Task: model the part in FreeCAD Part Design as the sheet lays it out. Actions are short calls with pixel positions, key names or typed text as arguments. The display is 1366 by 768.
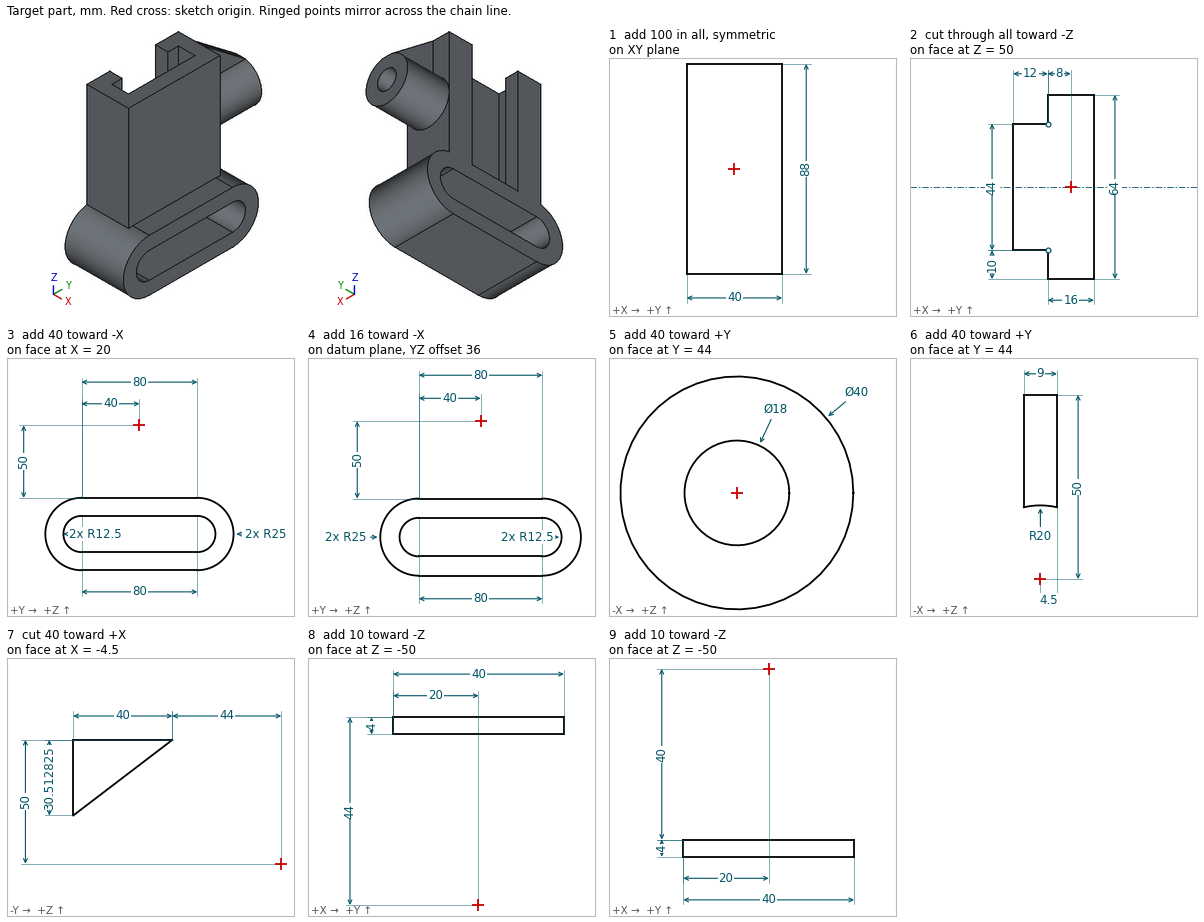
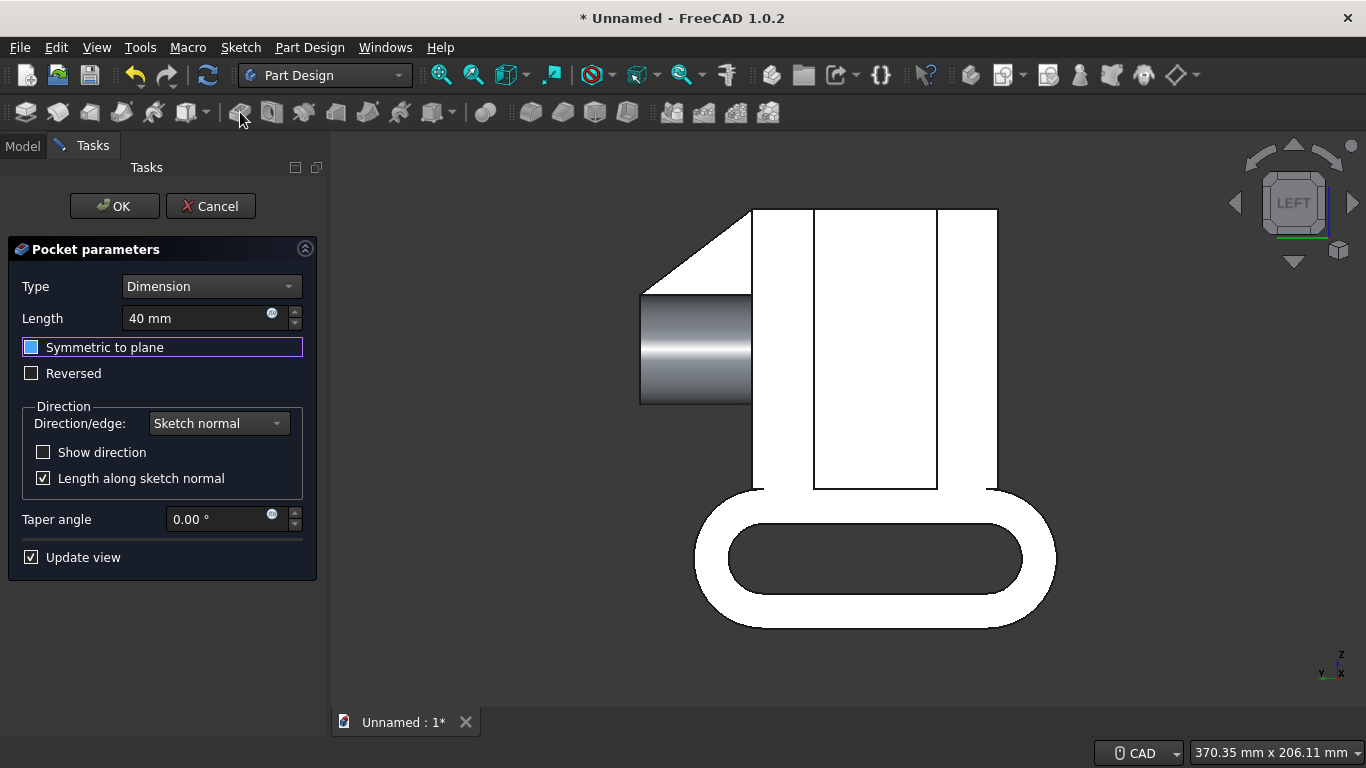
click(115, 206)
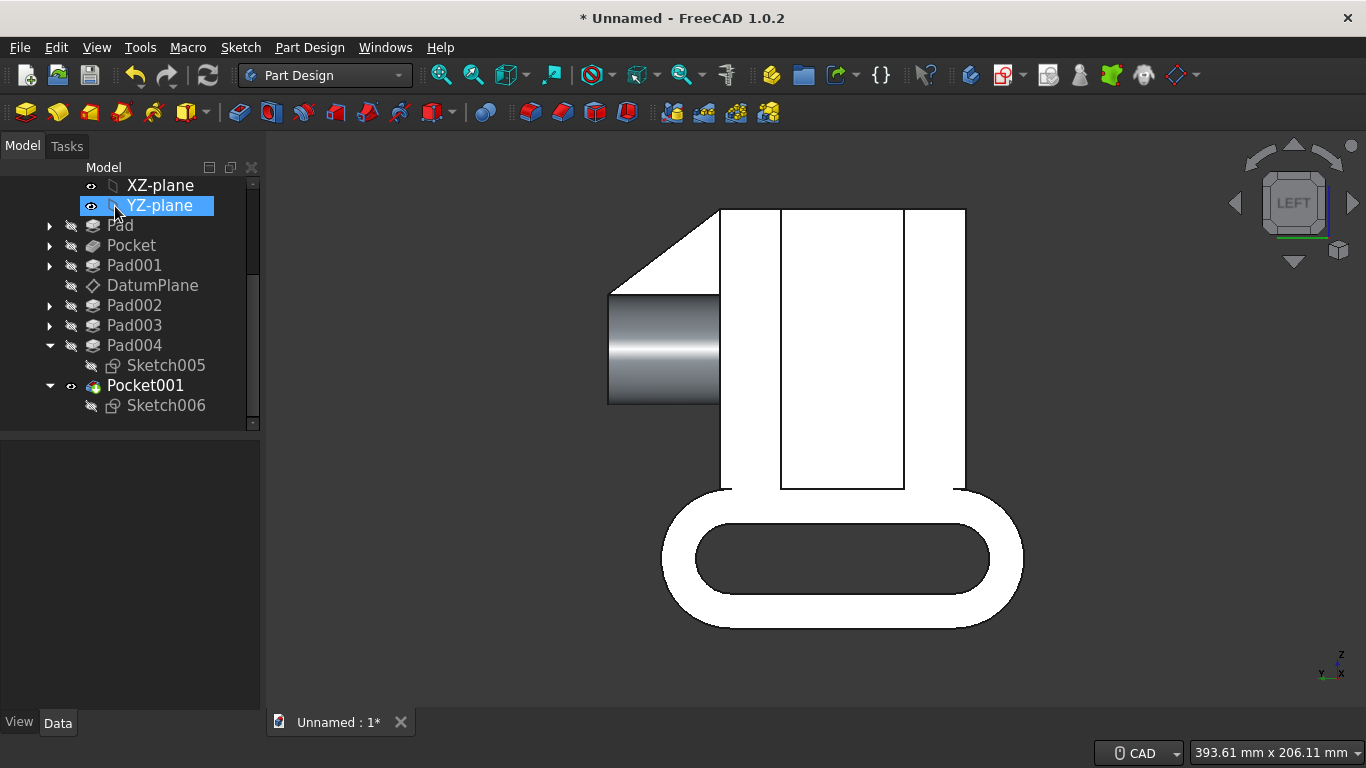
key(0)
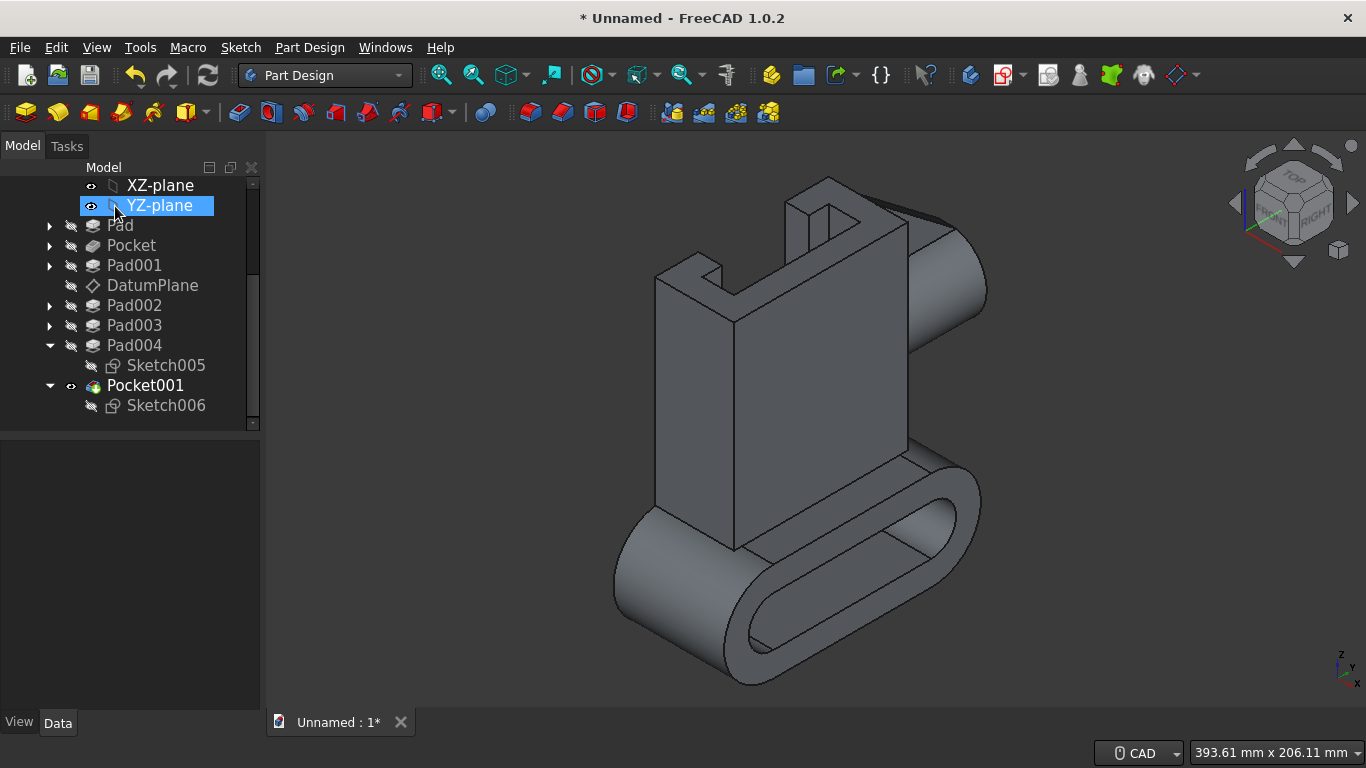
key(v)
key(f)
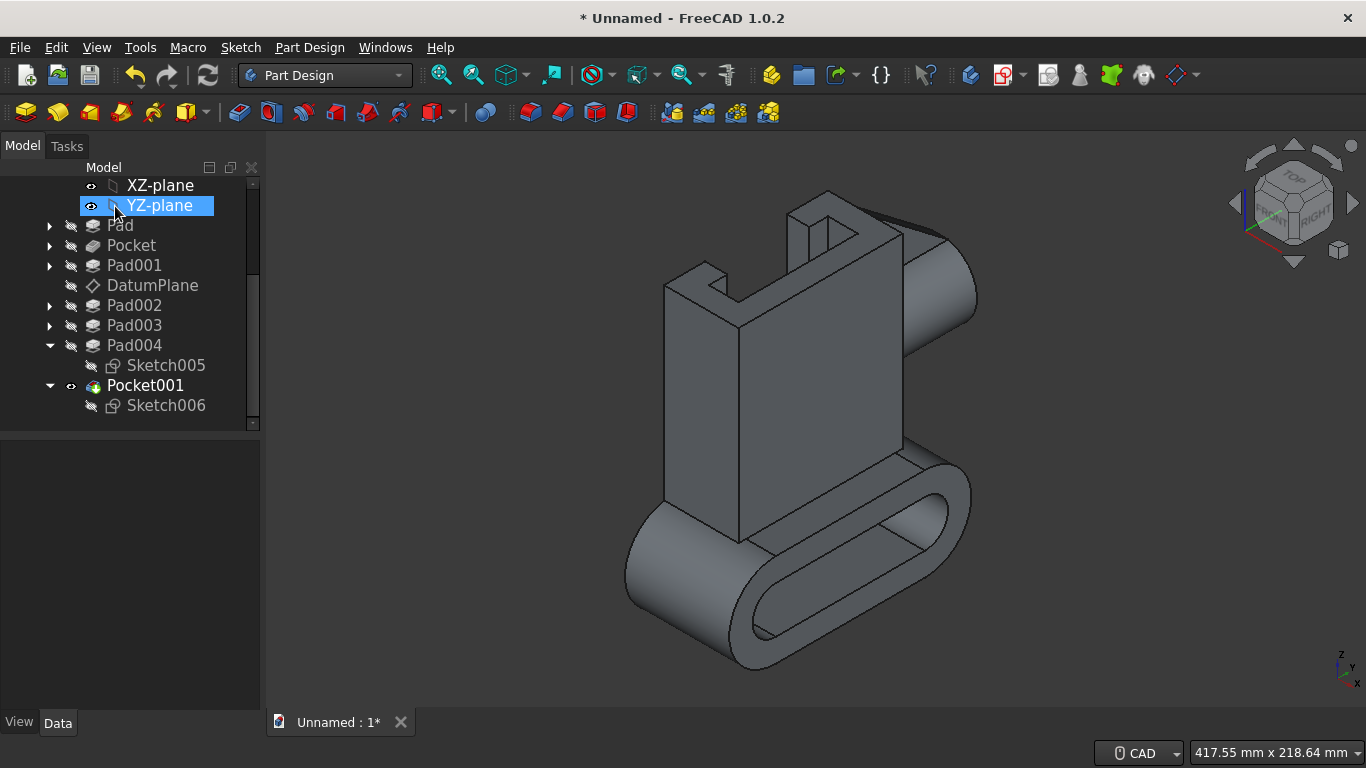
key(2)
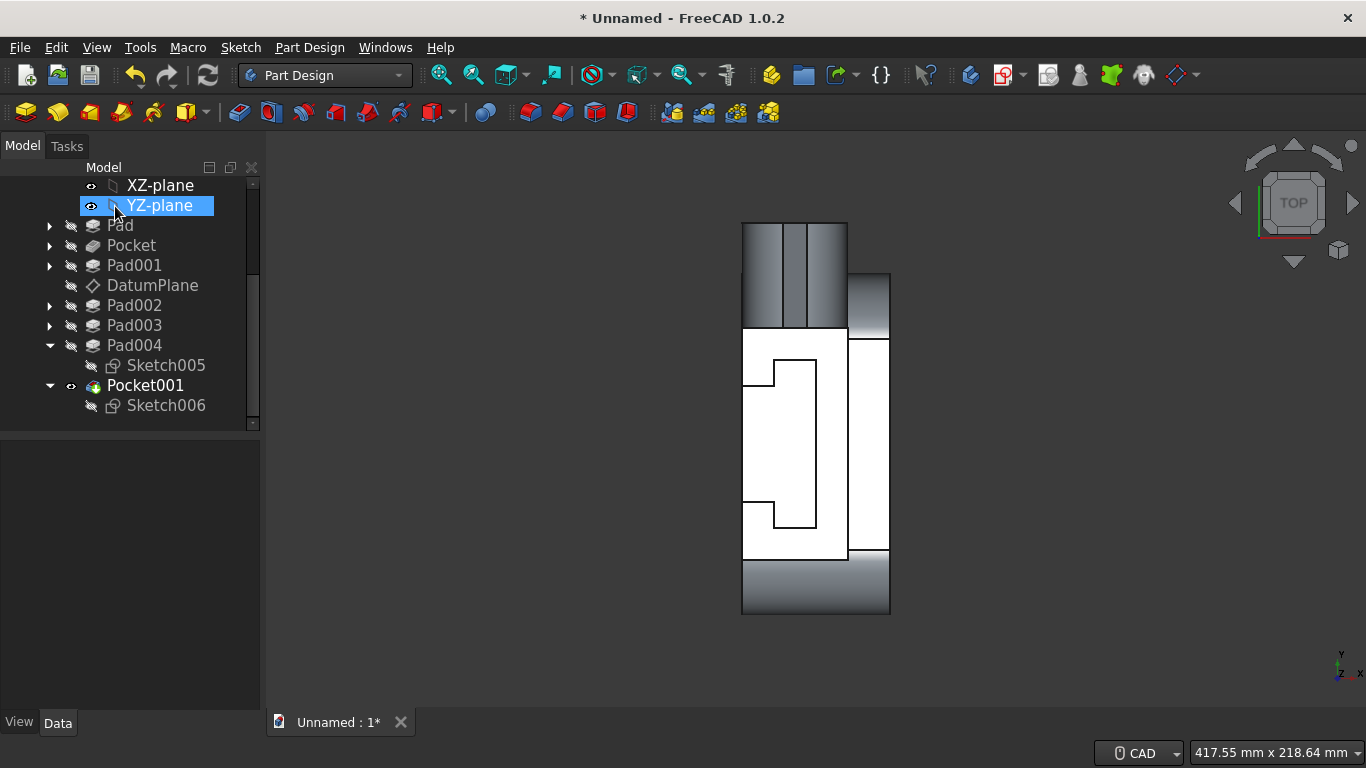
click(779, 443)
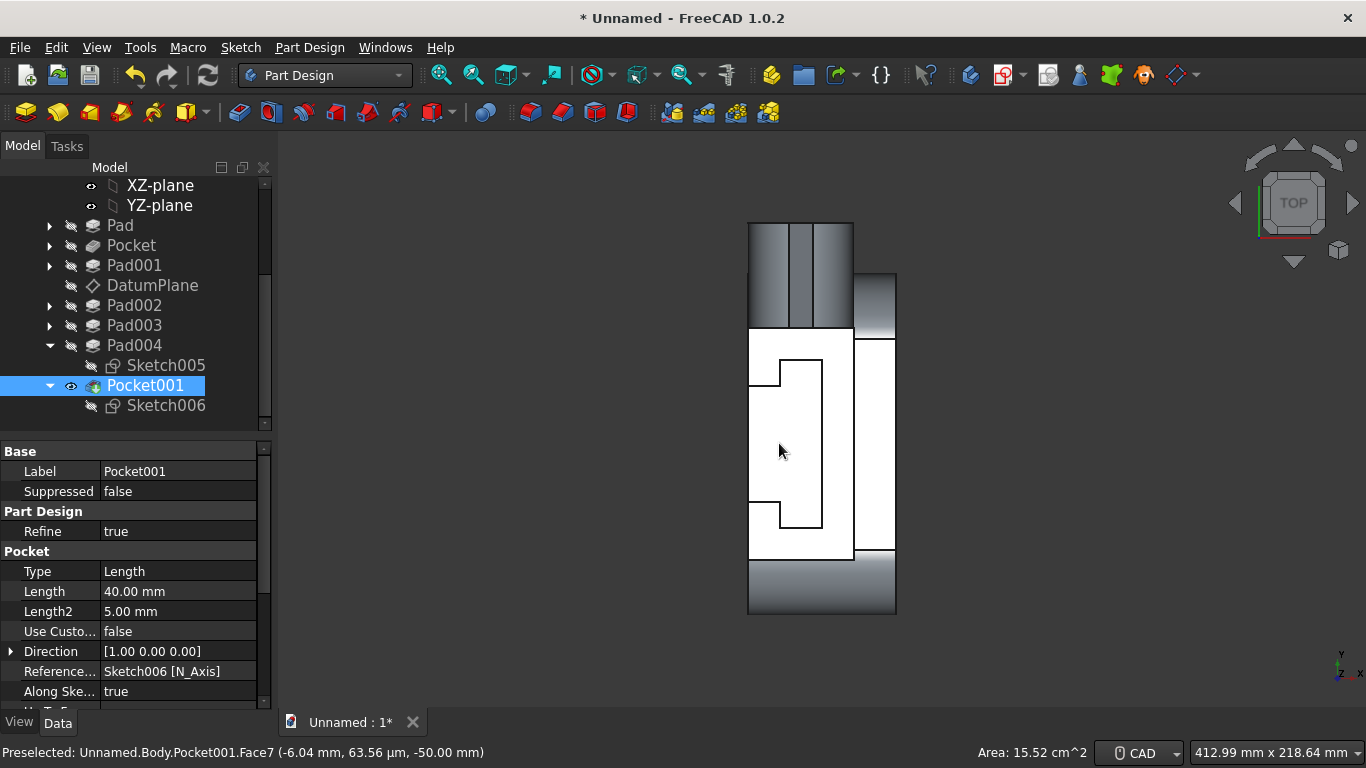
click(1004, 76)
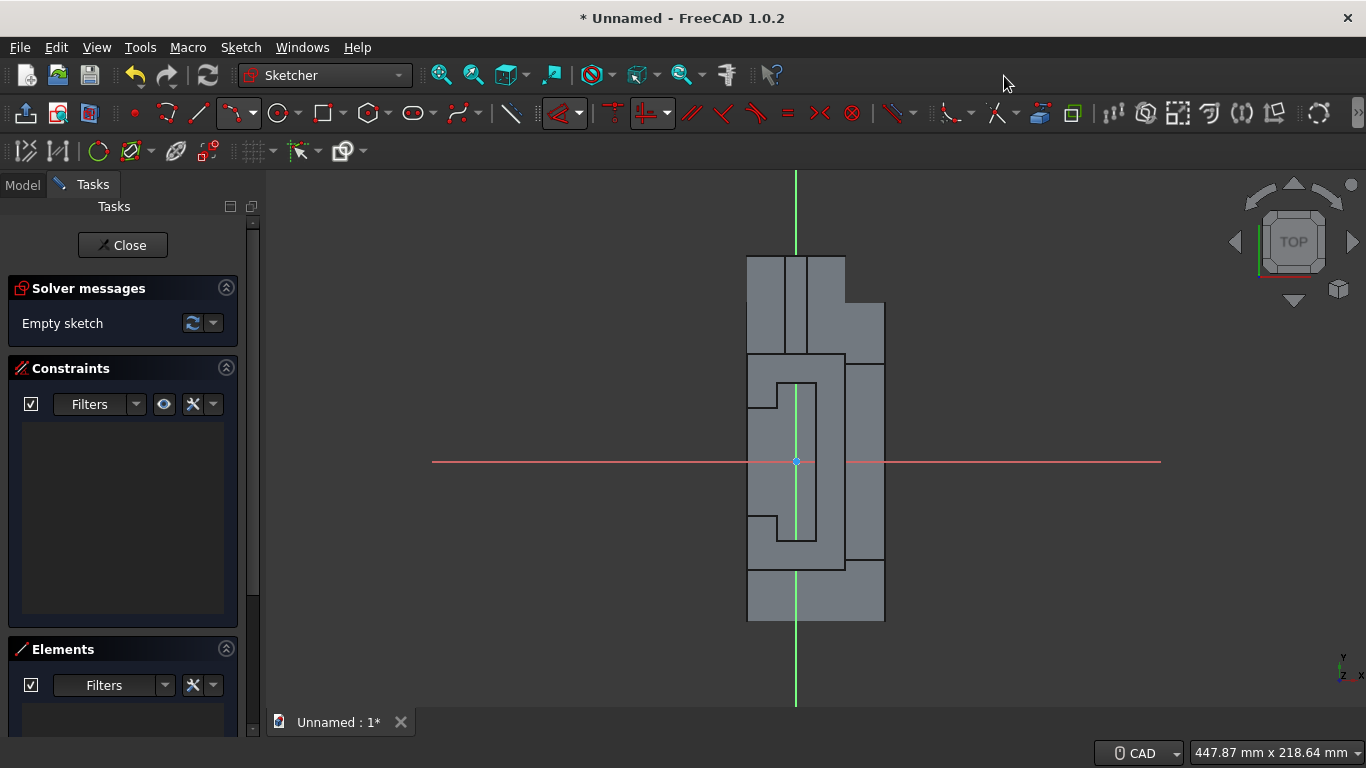
scroll(817, 395, up, 6)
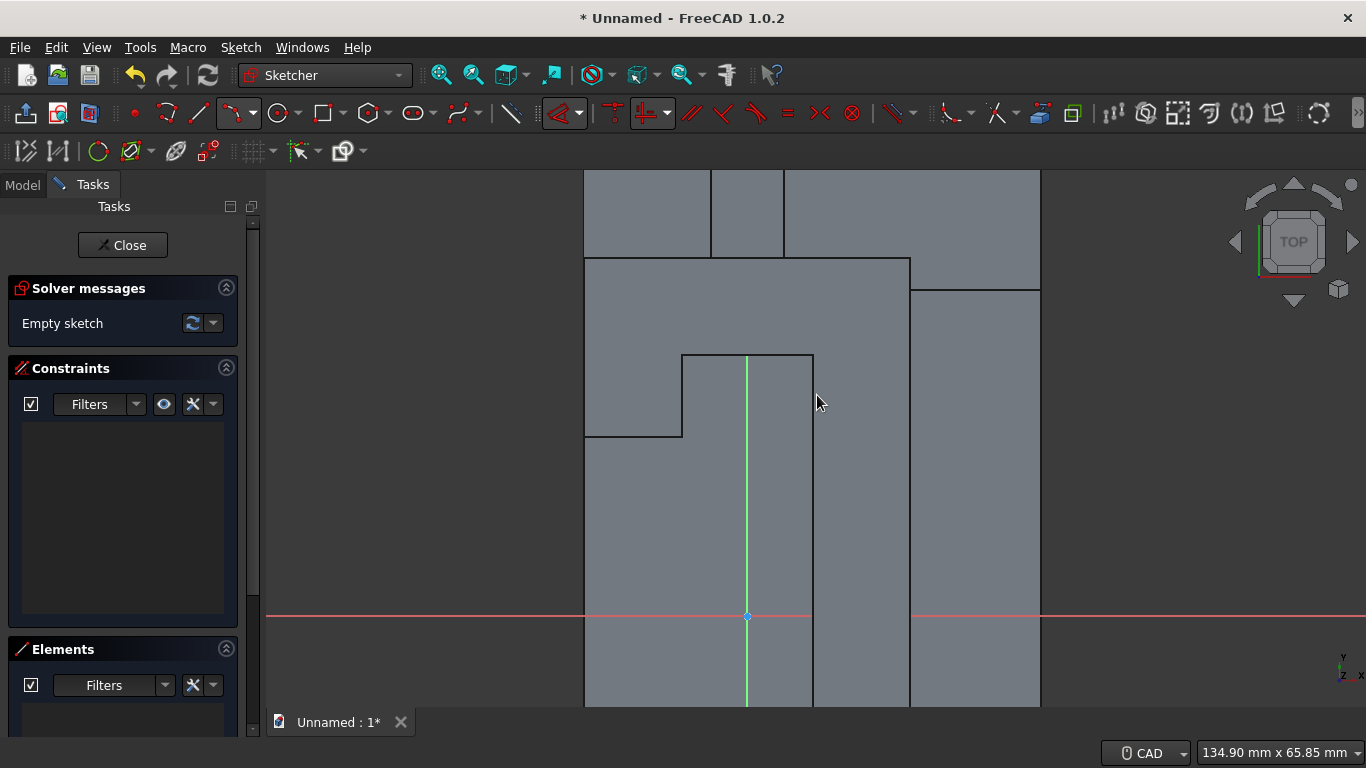
key(g)
key(r)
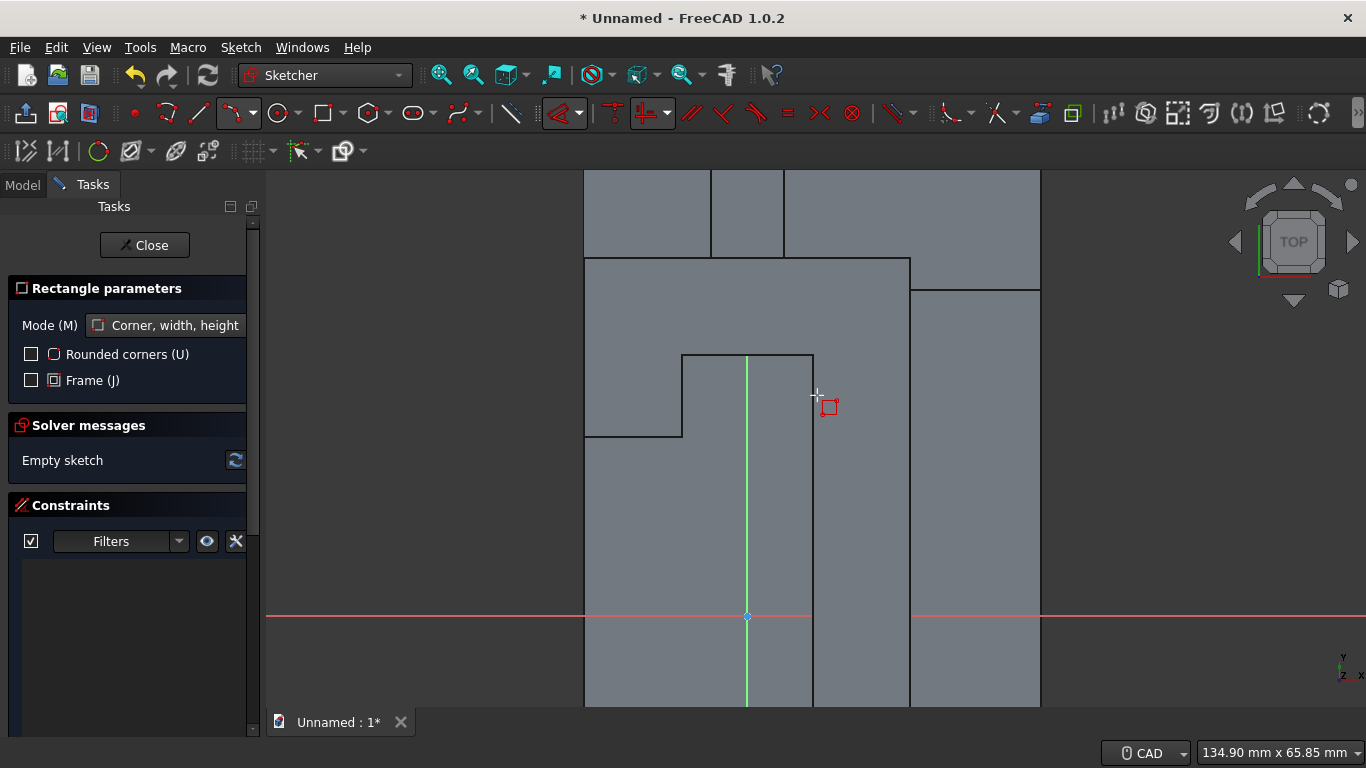
click(584, 258)
click(910, 290)
key(Escape)